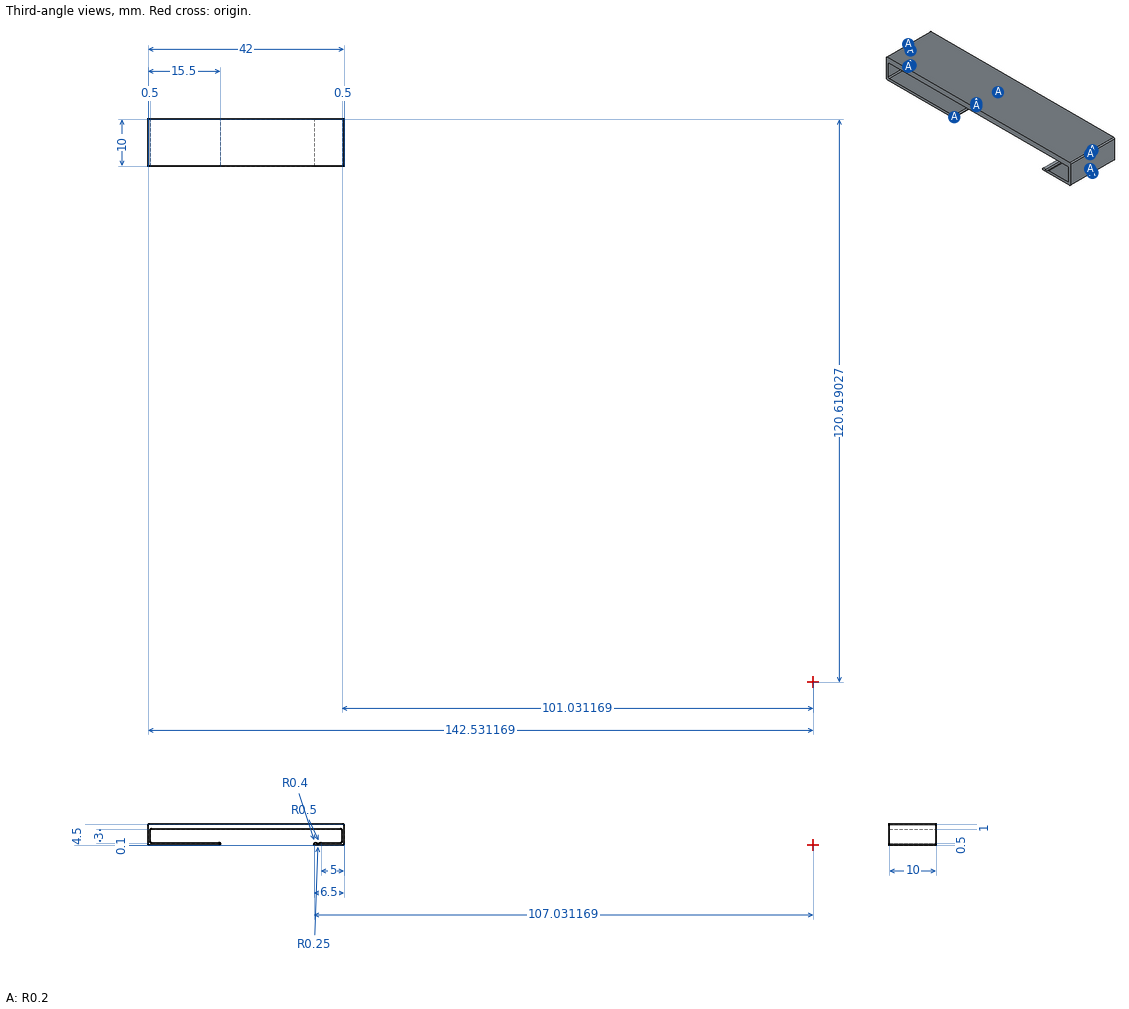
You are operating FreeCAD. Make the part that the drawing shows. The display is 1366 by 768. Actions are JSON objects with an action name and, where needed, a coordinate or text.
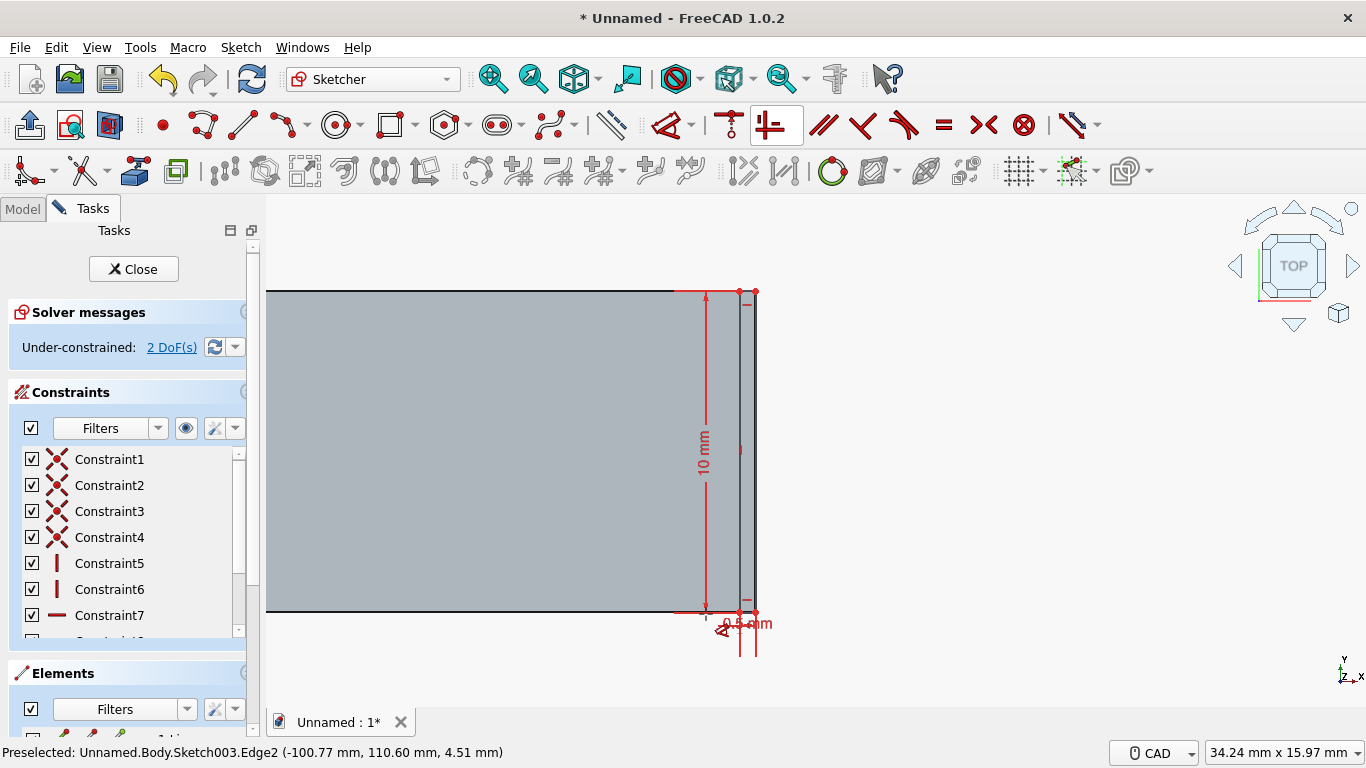
{"action": "left_click", "coordinate": [740, 291]}
{"action": "left_click", "coordinate": [970, 257]}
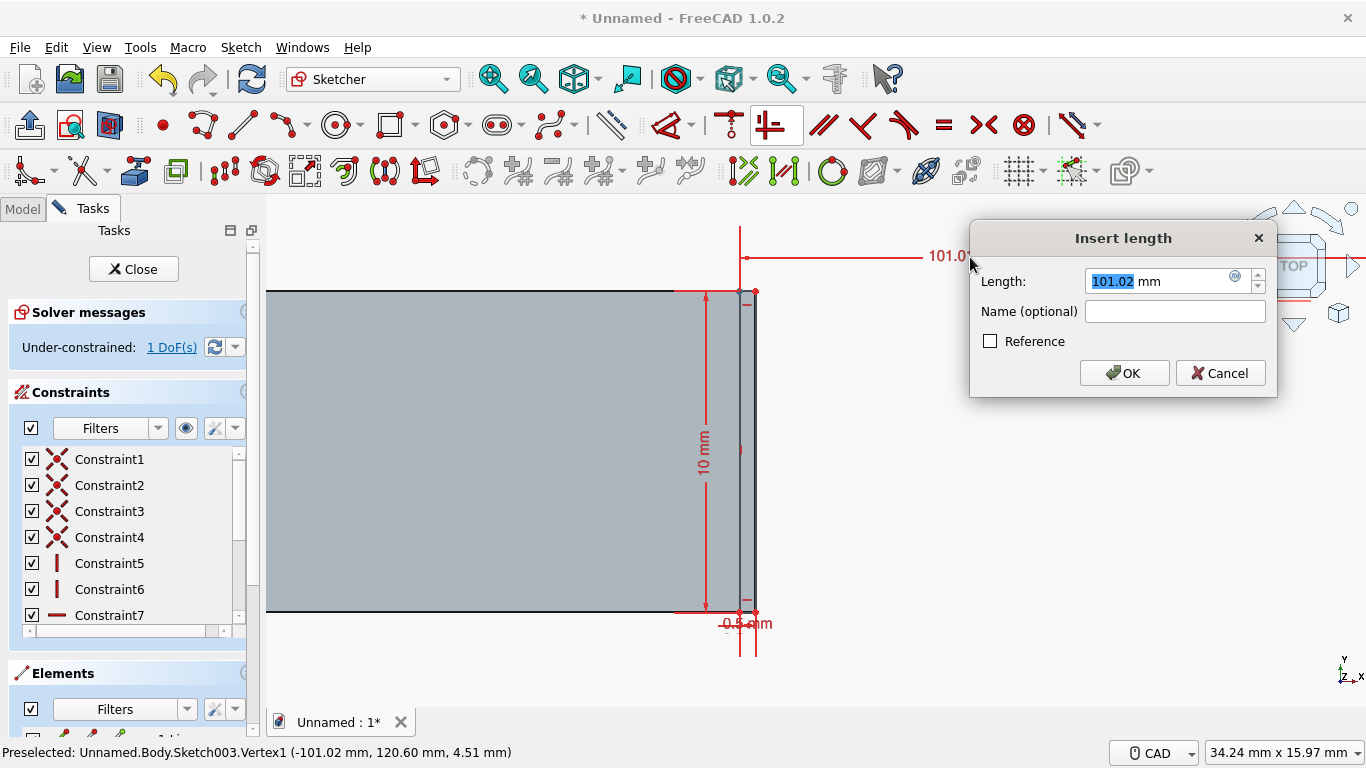
{"action": "type", "text": "101.031169"}
{"action": "key", "text": "Return"}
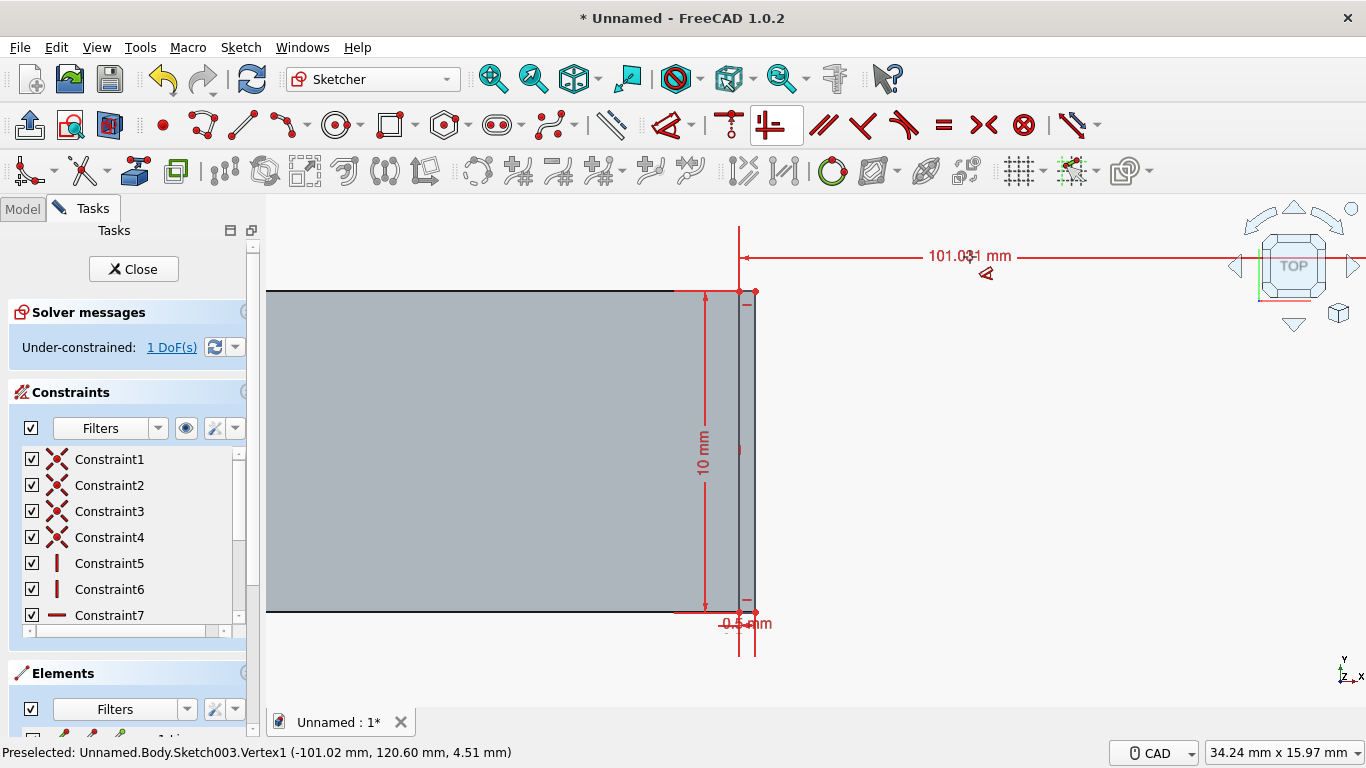
{"action": "left_click", "coordinate": [739, 291]}
{"action": "left_click", "coordinate": [705, 485]}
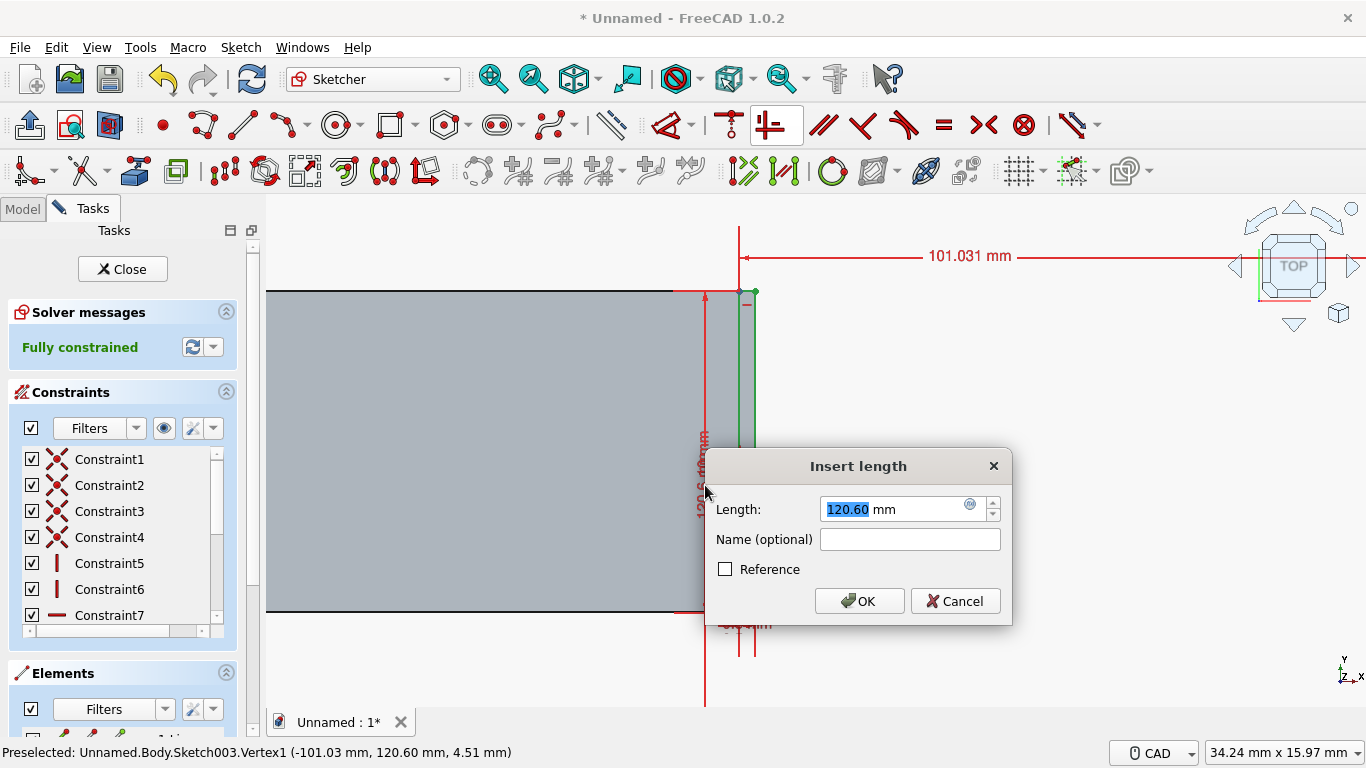
{"action": "type", "text": "120.619027"}
{"action": "key", "text": "Return"}
{"action": "key", "text": "Escape"}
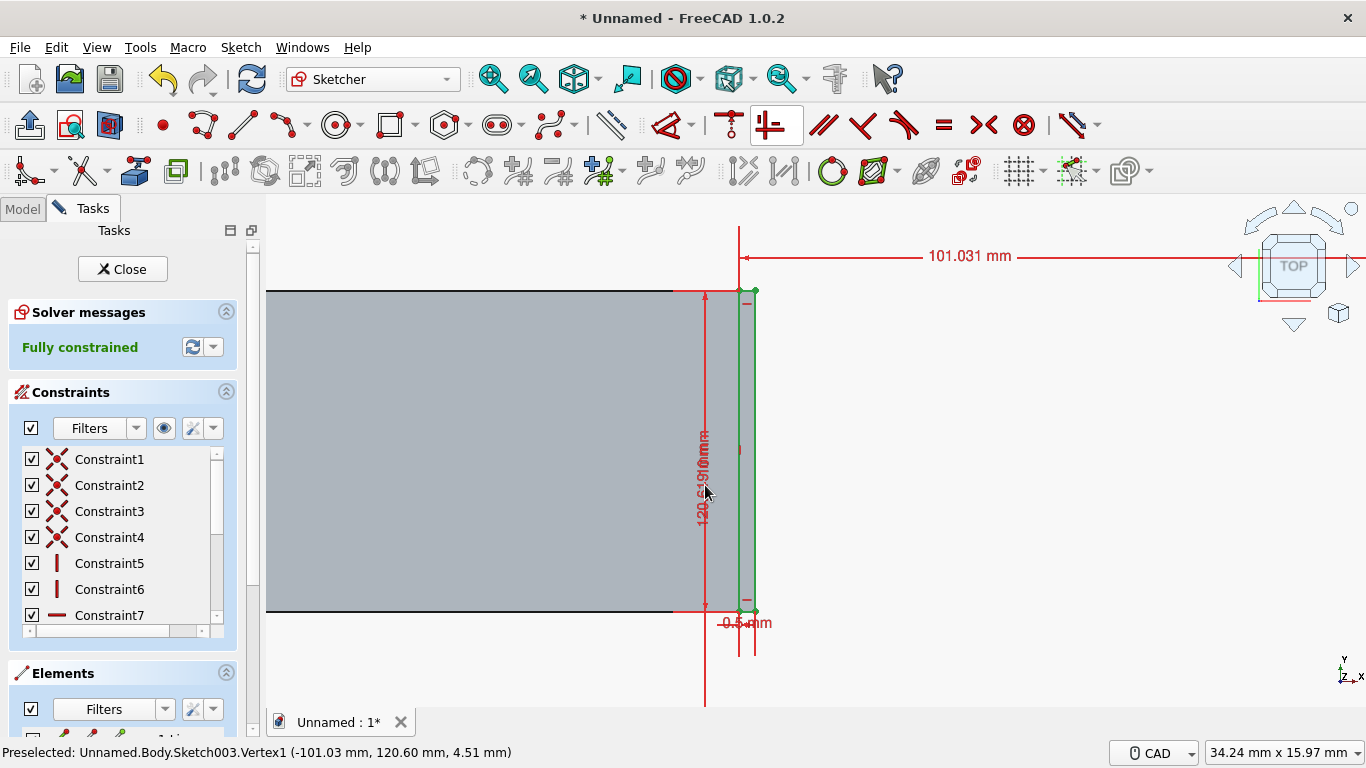
{"action": "left_click", "coordinate": [123, 269]}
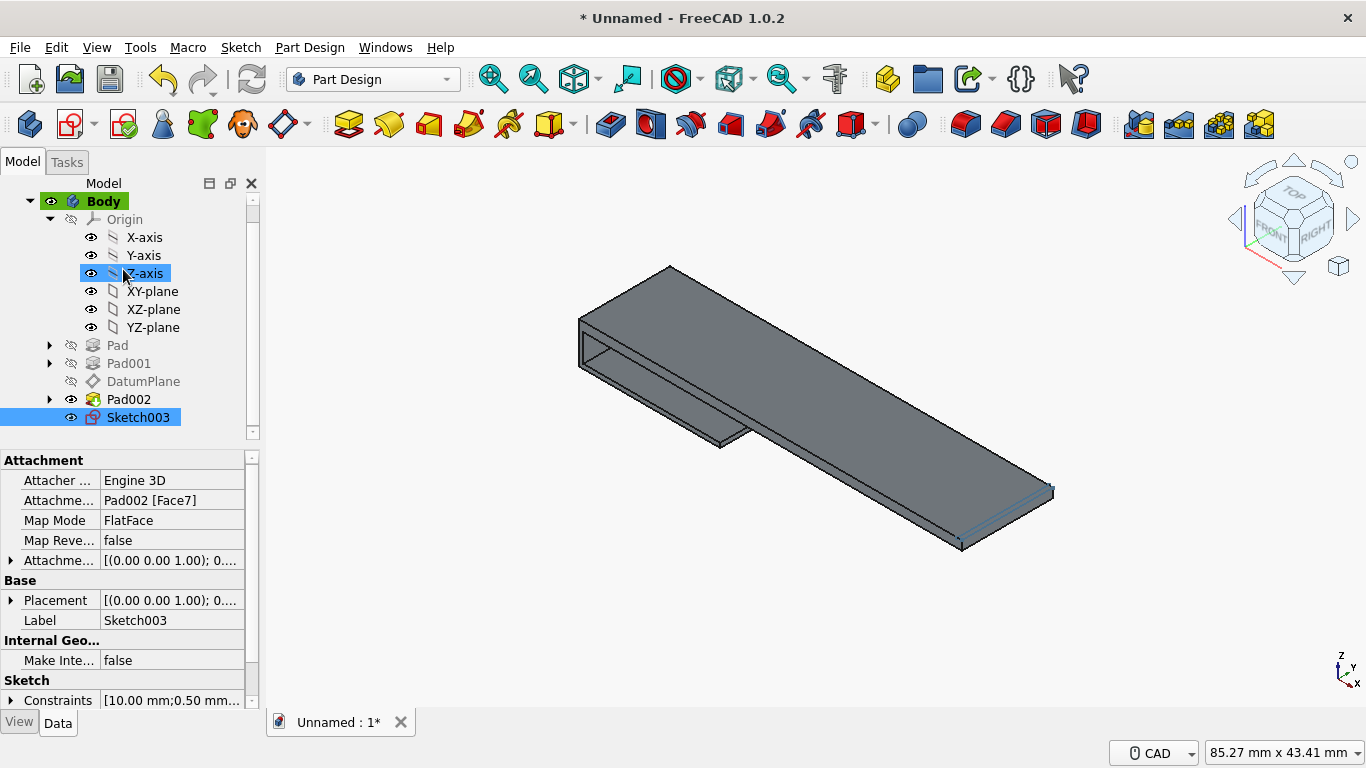
{"action": "left_click", "coordinate": [350, 124]}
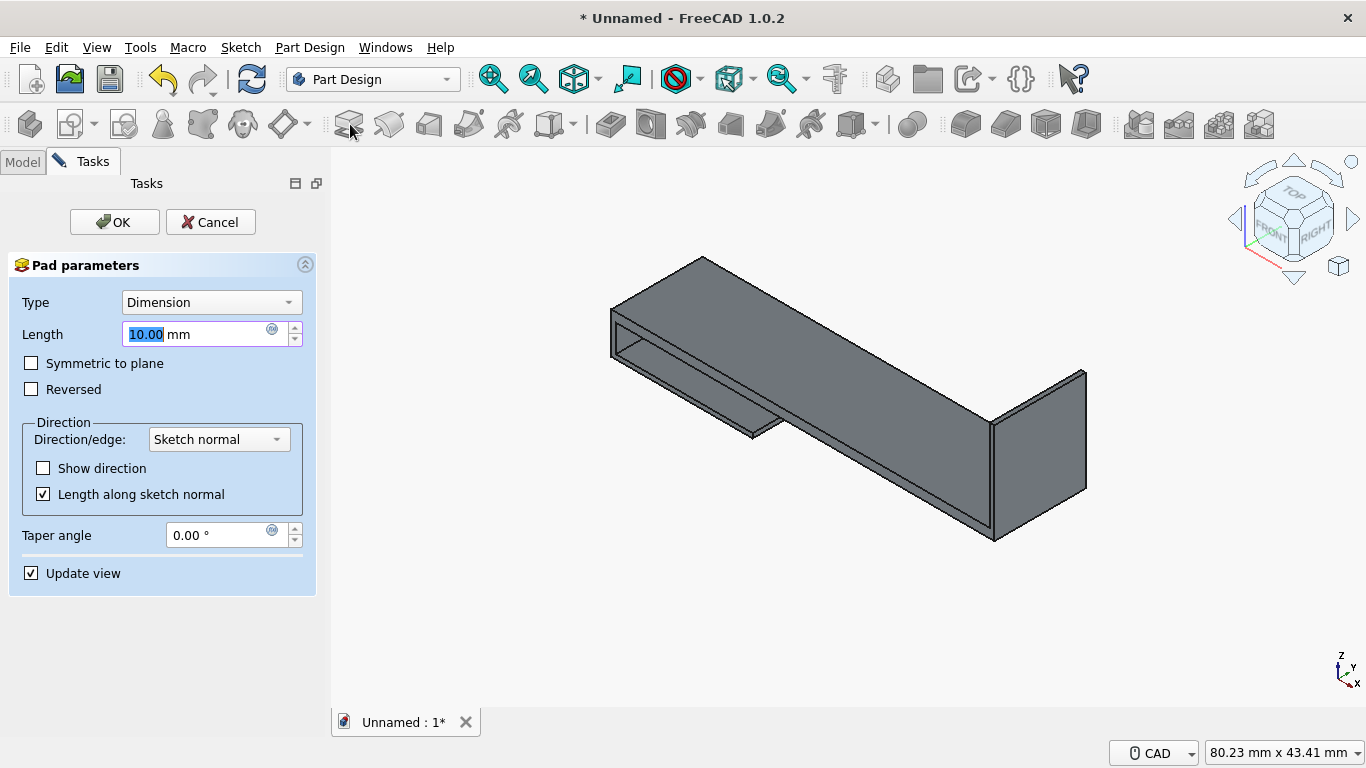
{"action": "type", "text": "4.5"}
{"action": "key", "text": "Tab"}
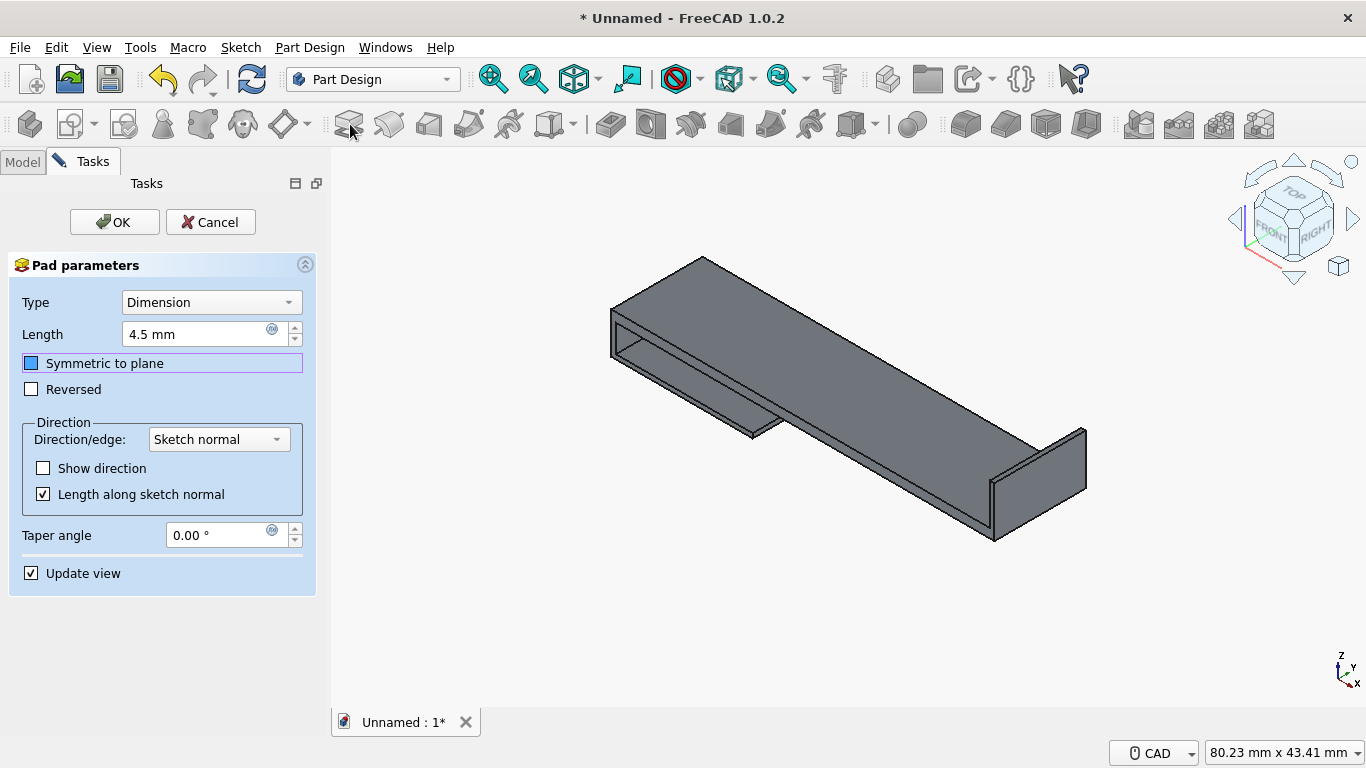
{"action": "left_click", "coordinate": [30, 389]}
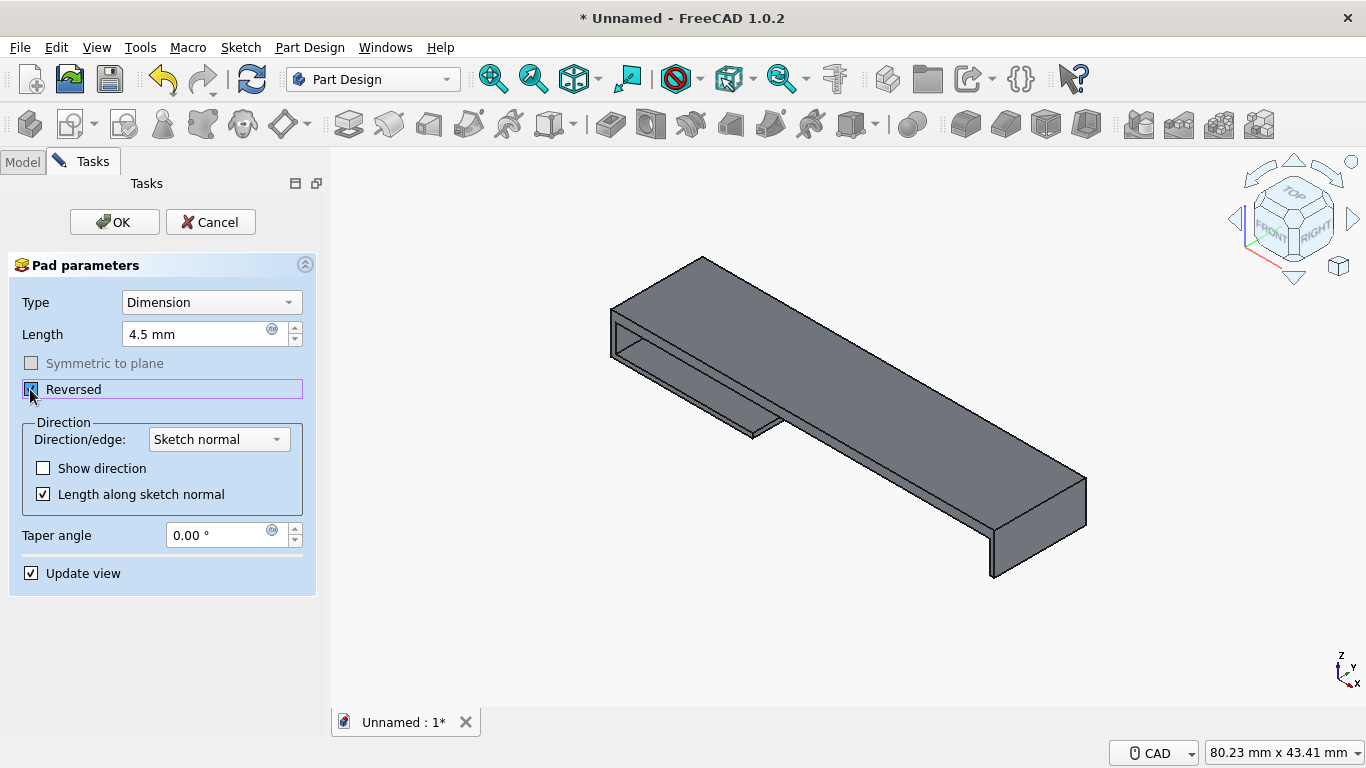
{"action": "left_click", "coordinate": [115, 222]}